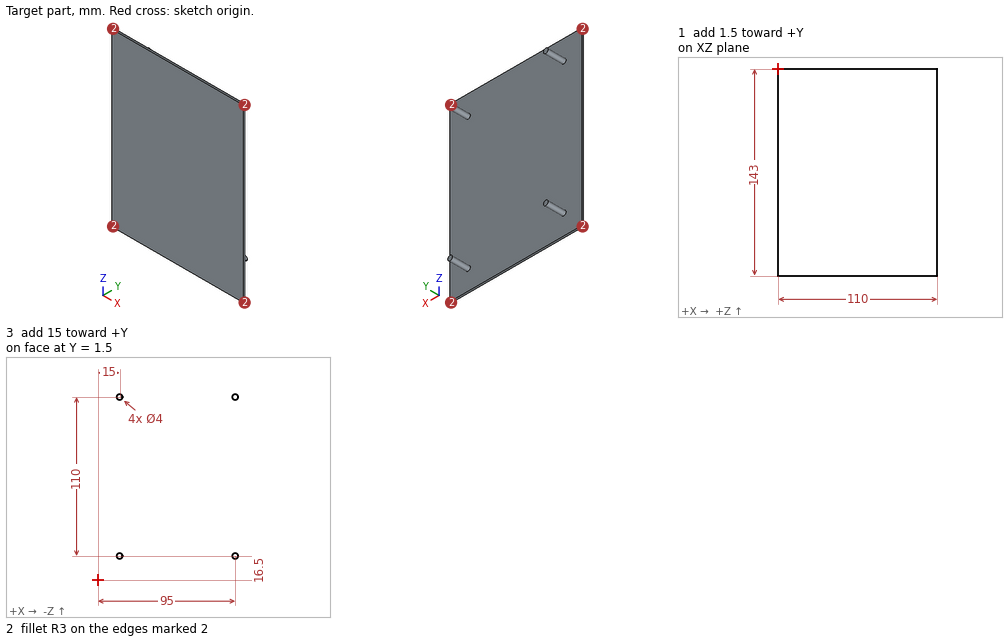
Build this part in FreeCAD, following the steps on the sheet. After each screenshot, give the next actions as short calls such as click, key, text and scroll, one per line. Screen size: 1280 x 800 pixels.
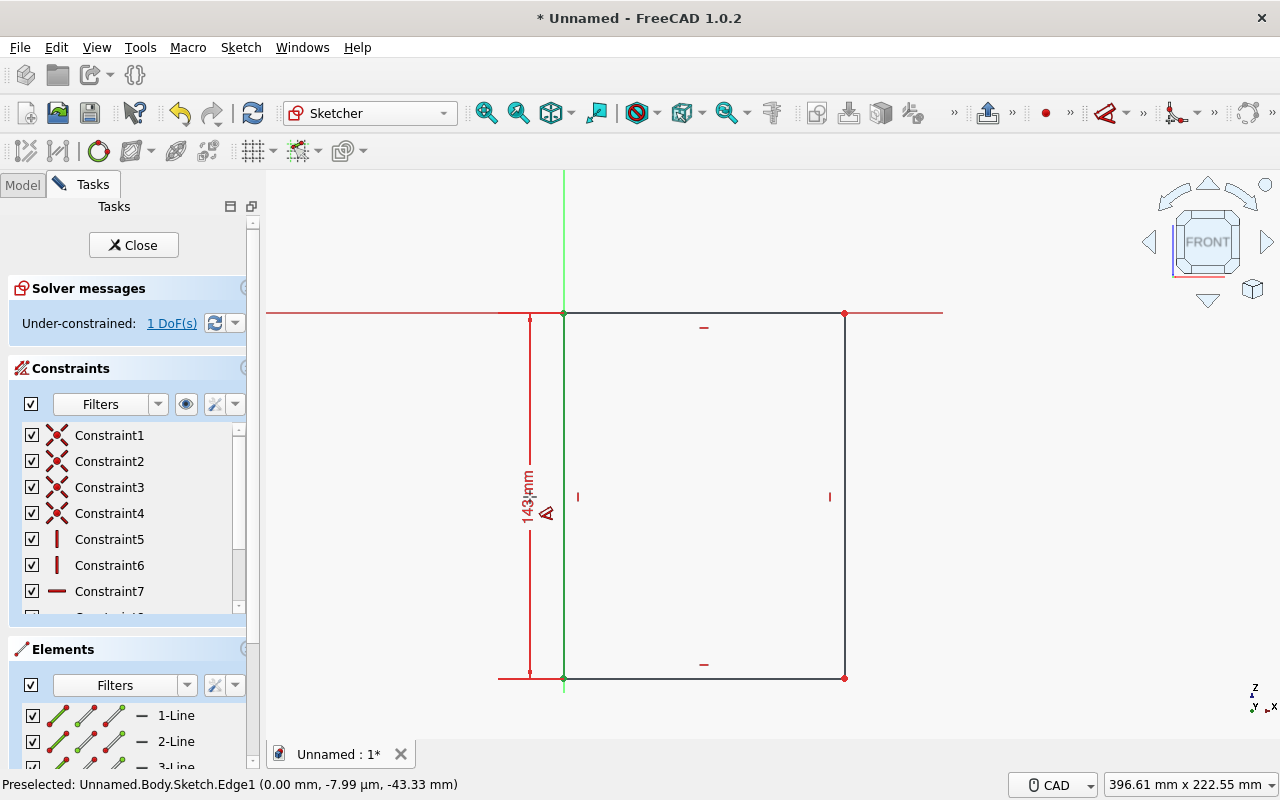
click(648, 679)
click(704, 645)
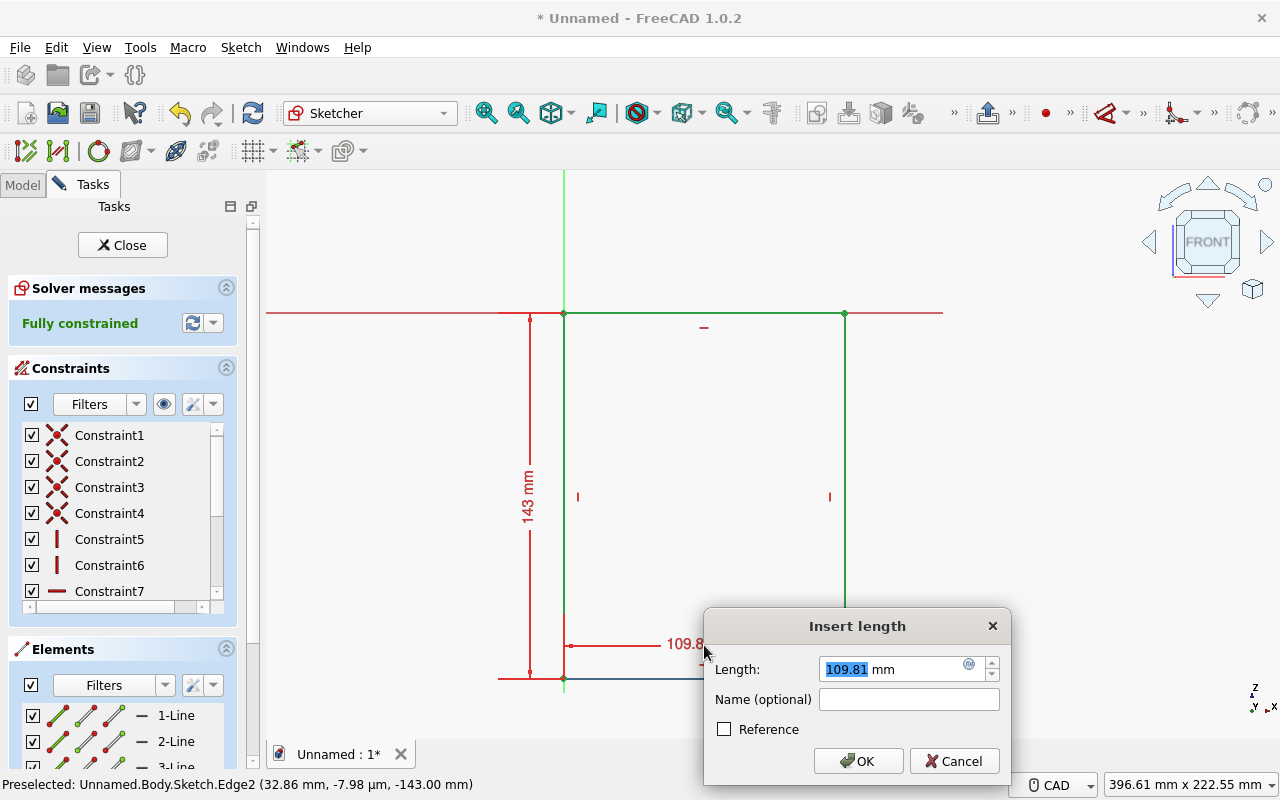
text(110)
key(Return)
key(Escape)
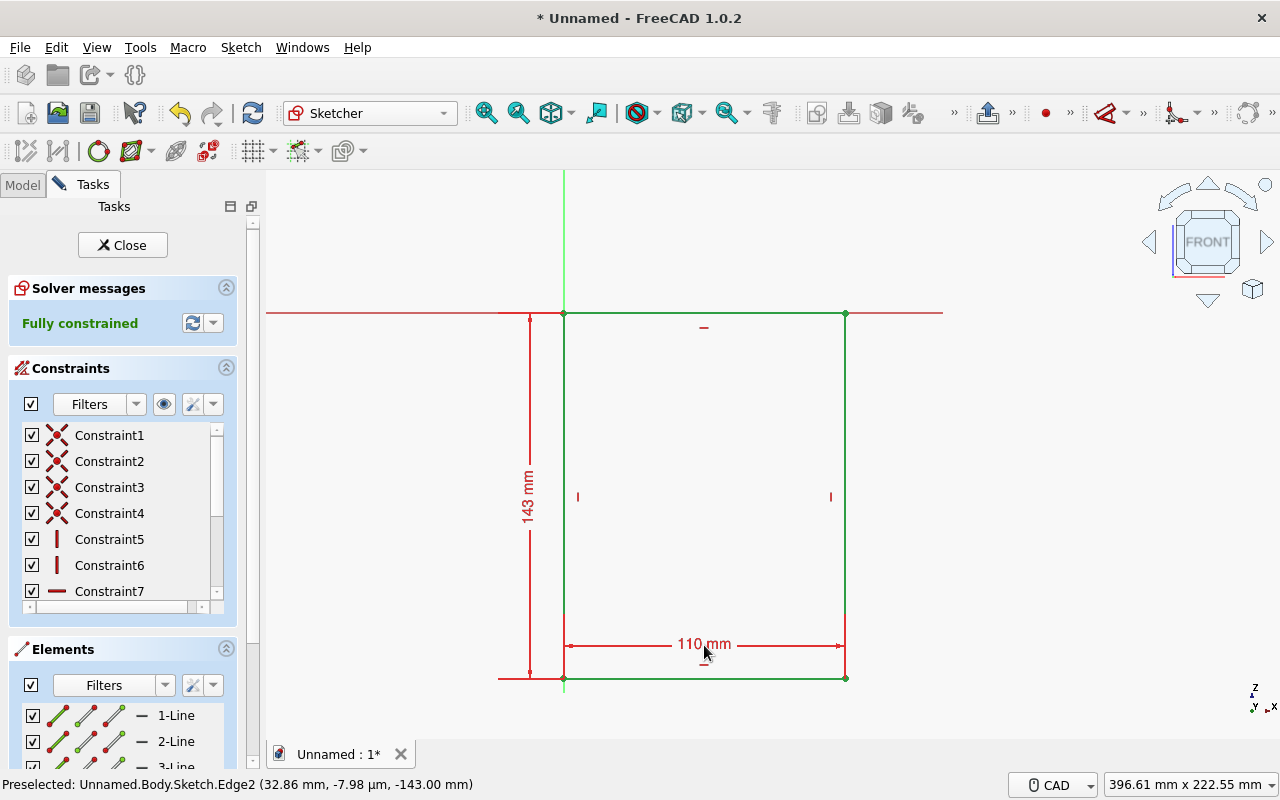
click(123, 245)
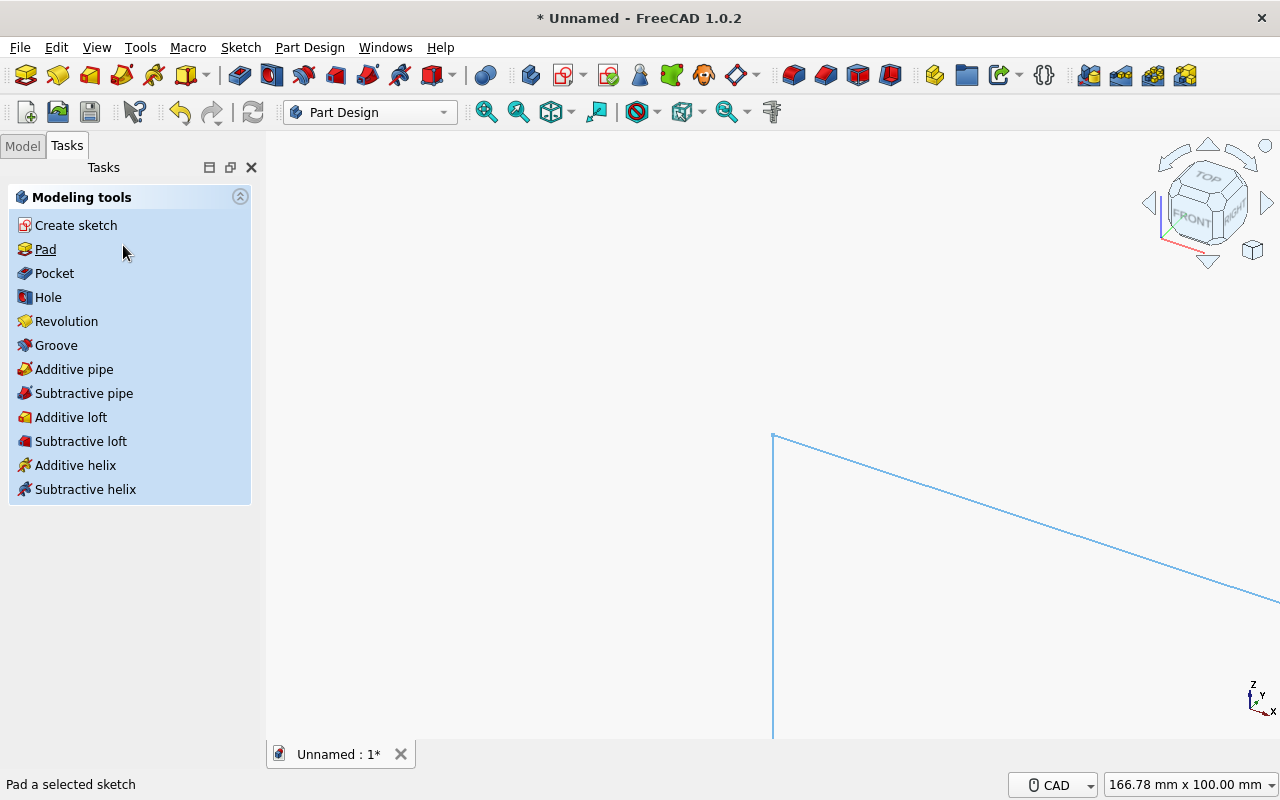
click(26, 76)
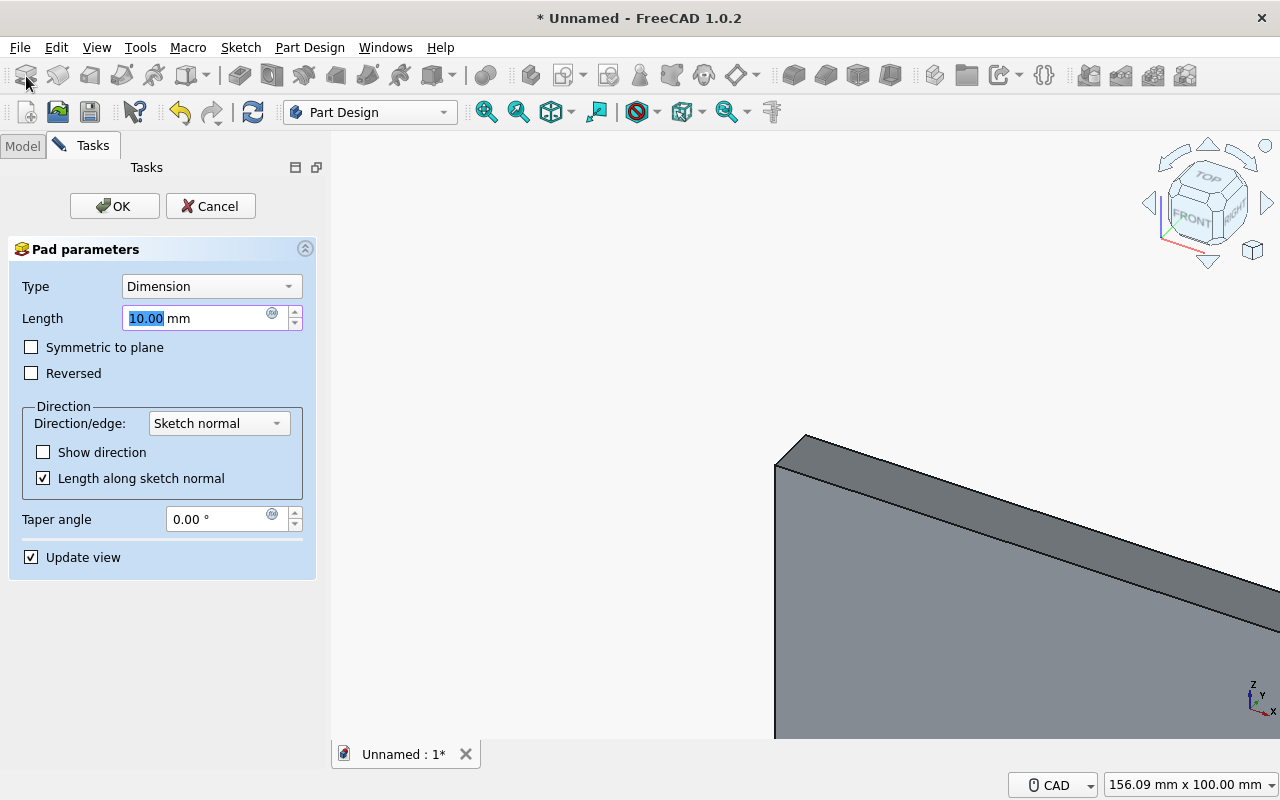
text(1.5)
key(Tab)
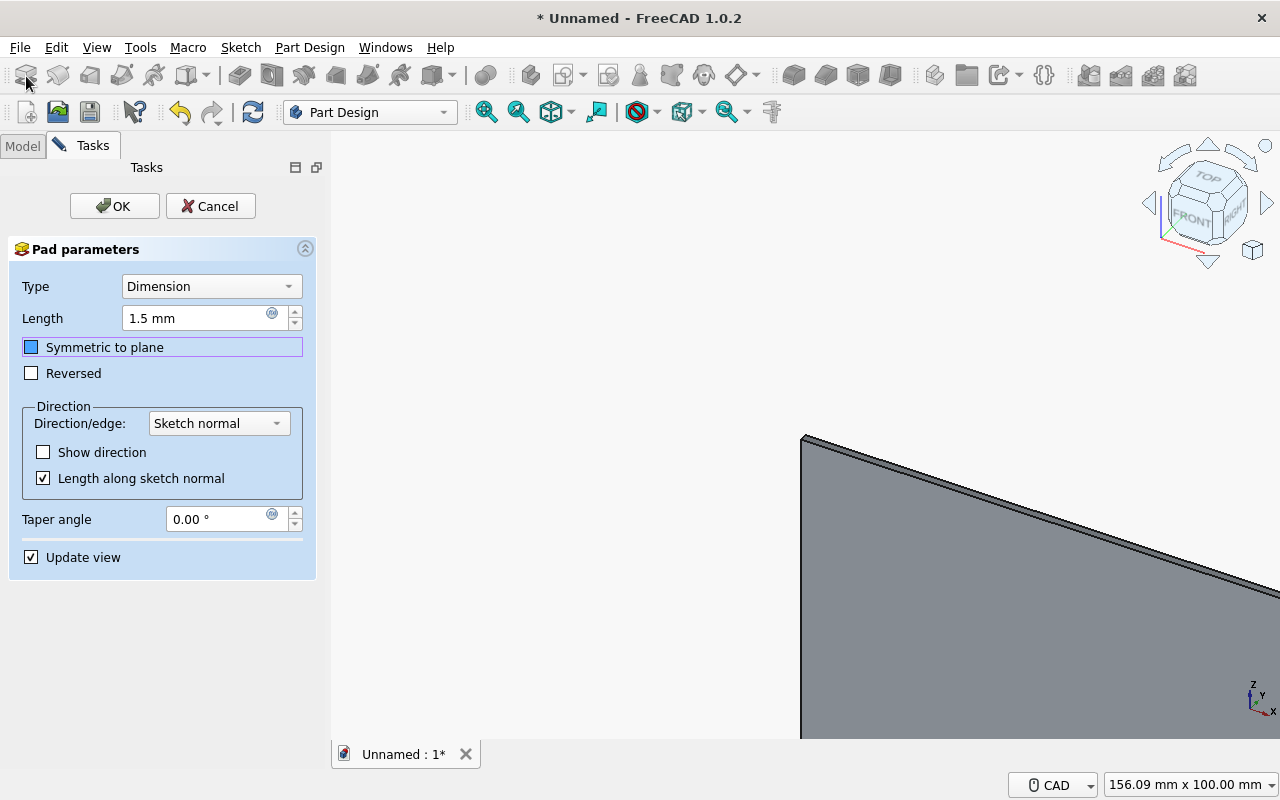
click(30, 373)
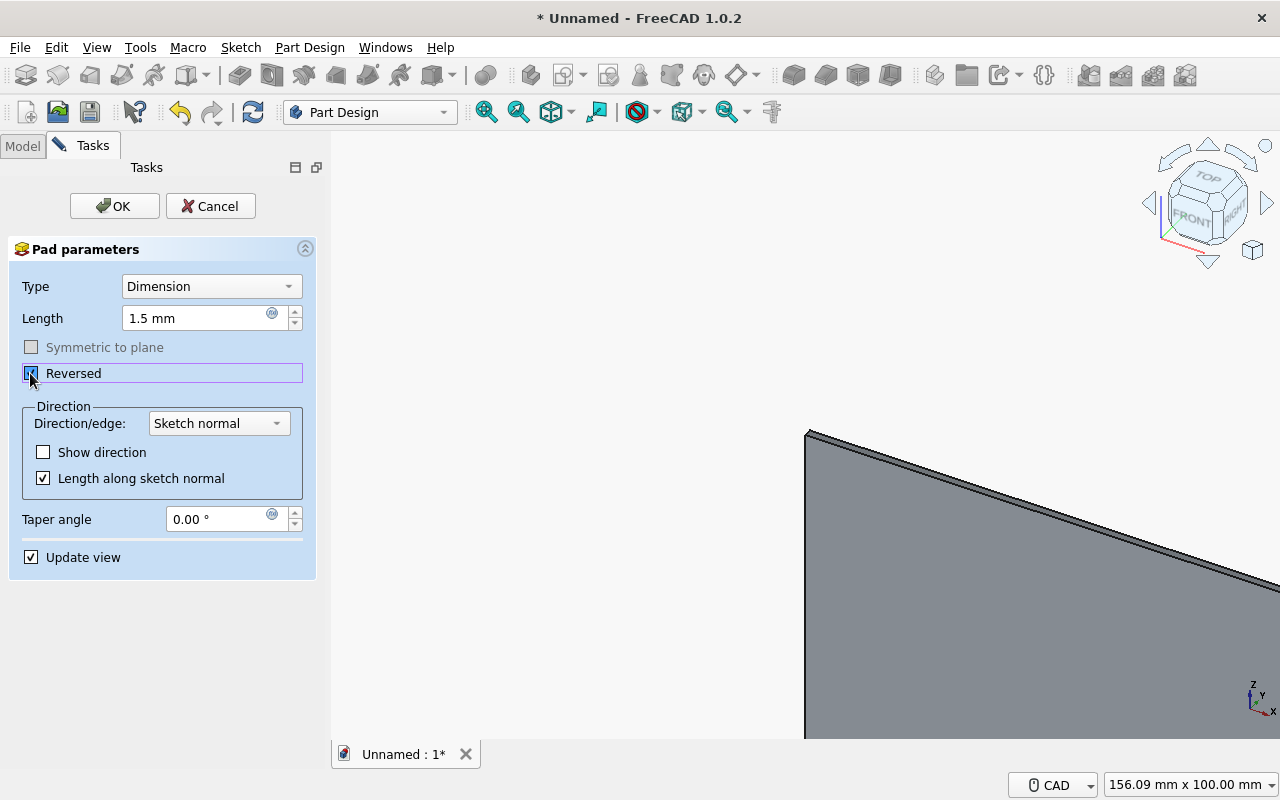
click(115, 206)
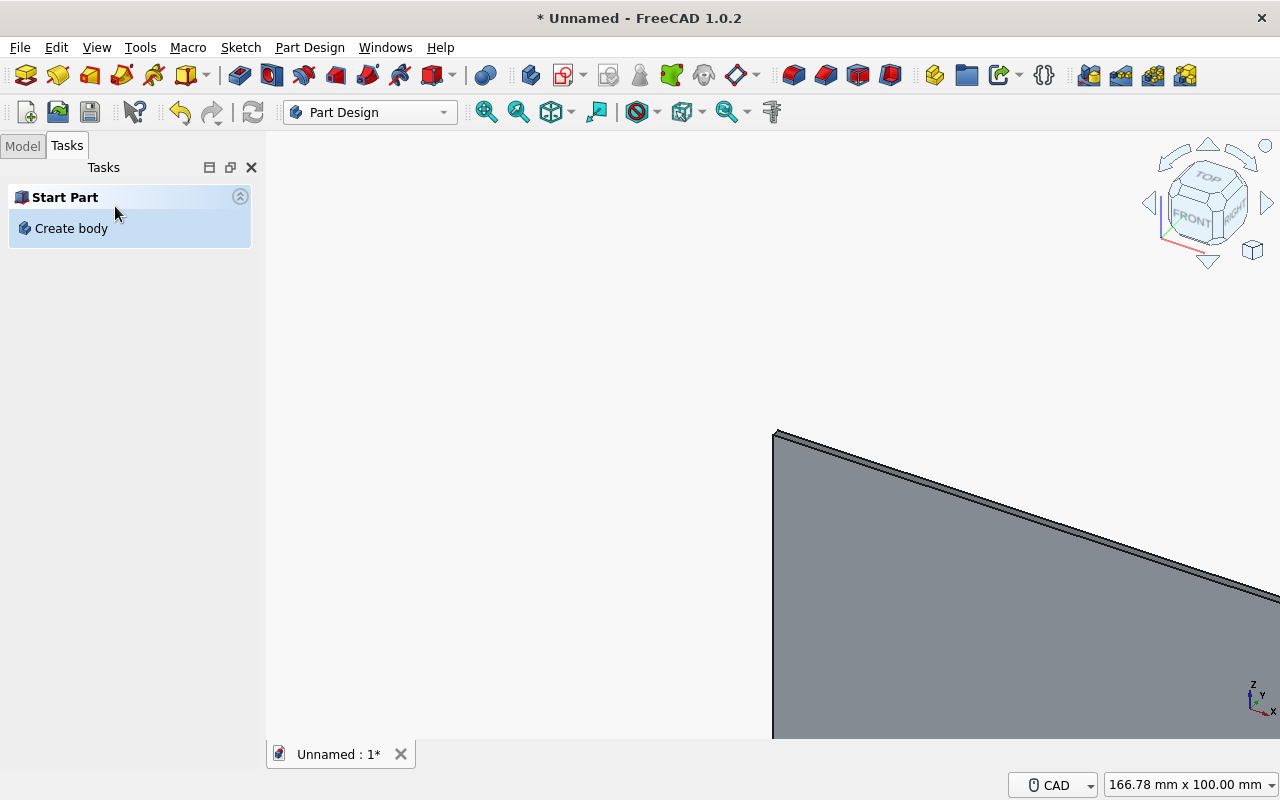
click(488, 112)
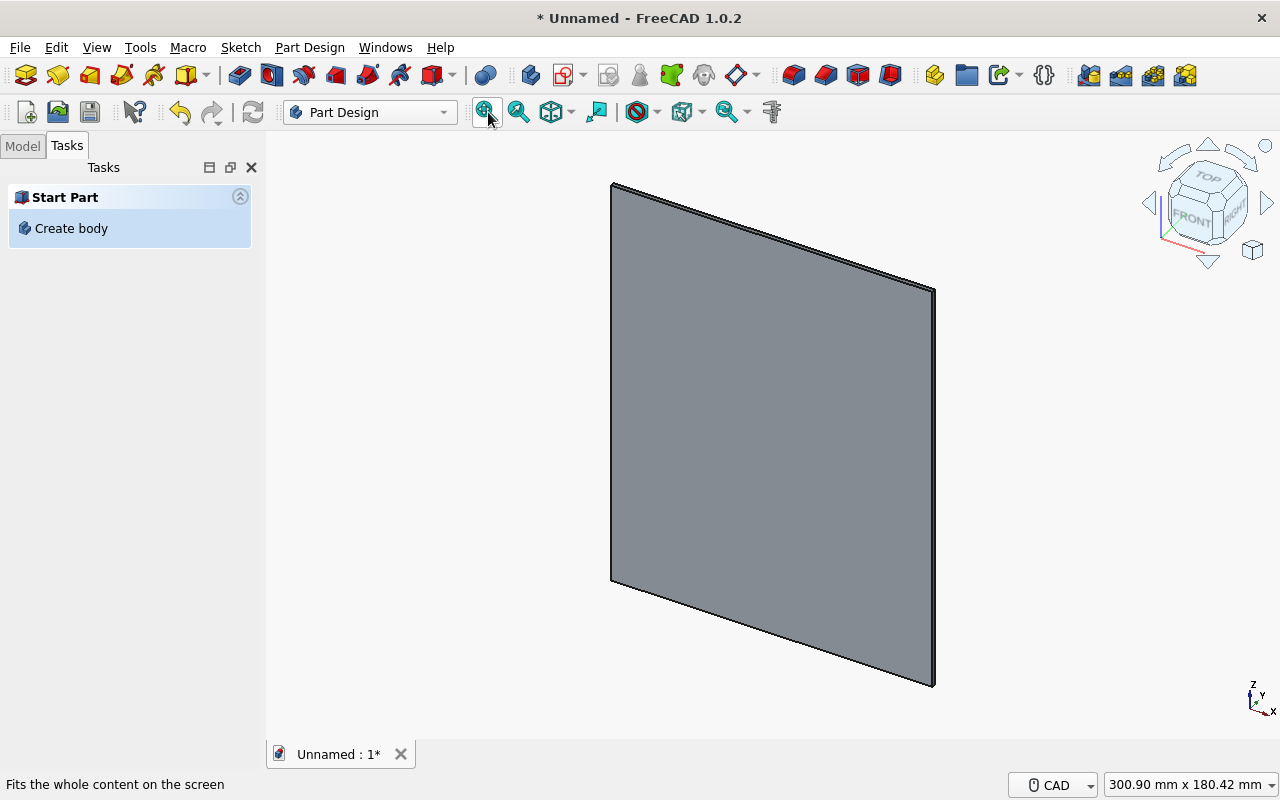
scroll(612, 578, up, 11)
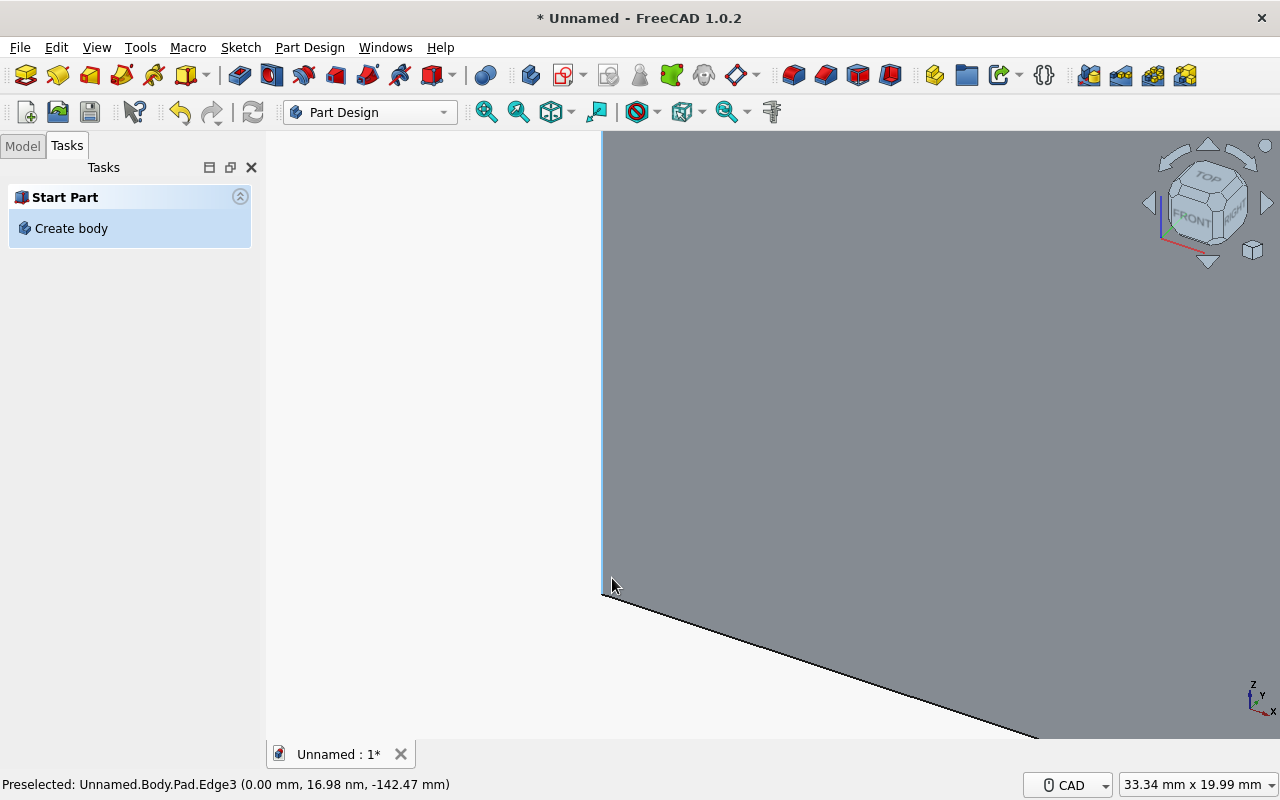
click(488, 112)